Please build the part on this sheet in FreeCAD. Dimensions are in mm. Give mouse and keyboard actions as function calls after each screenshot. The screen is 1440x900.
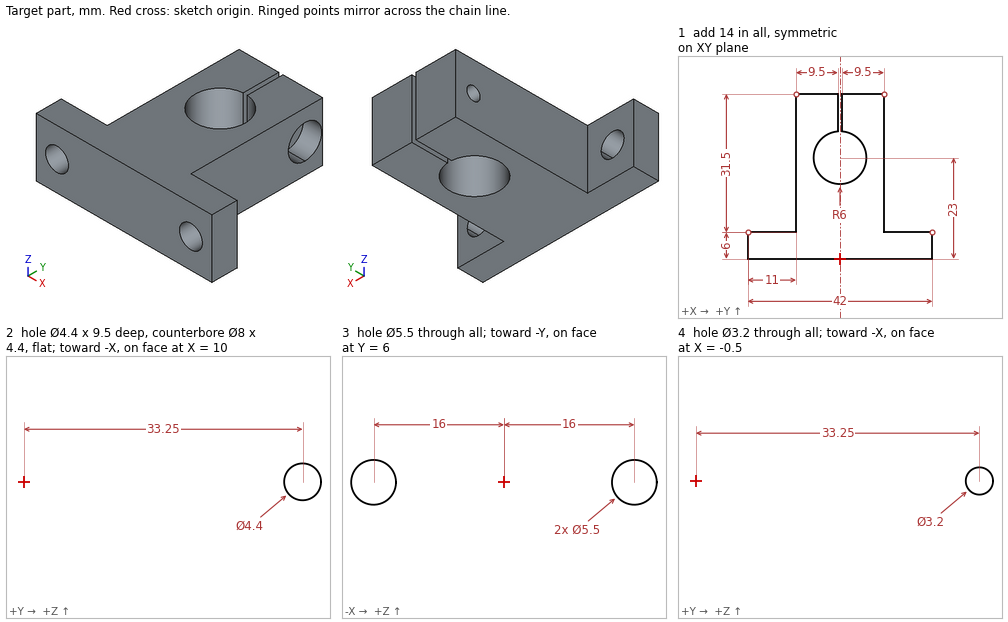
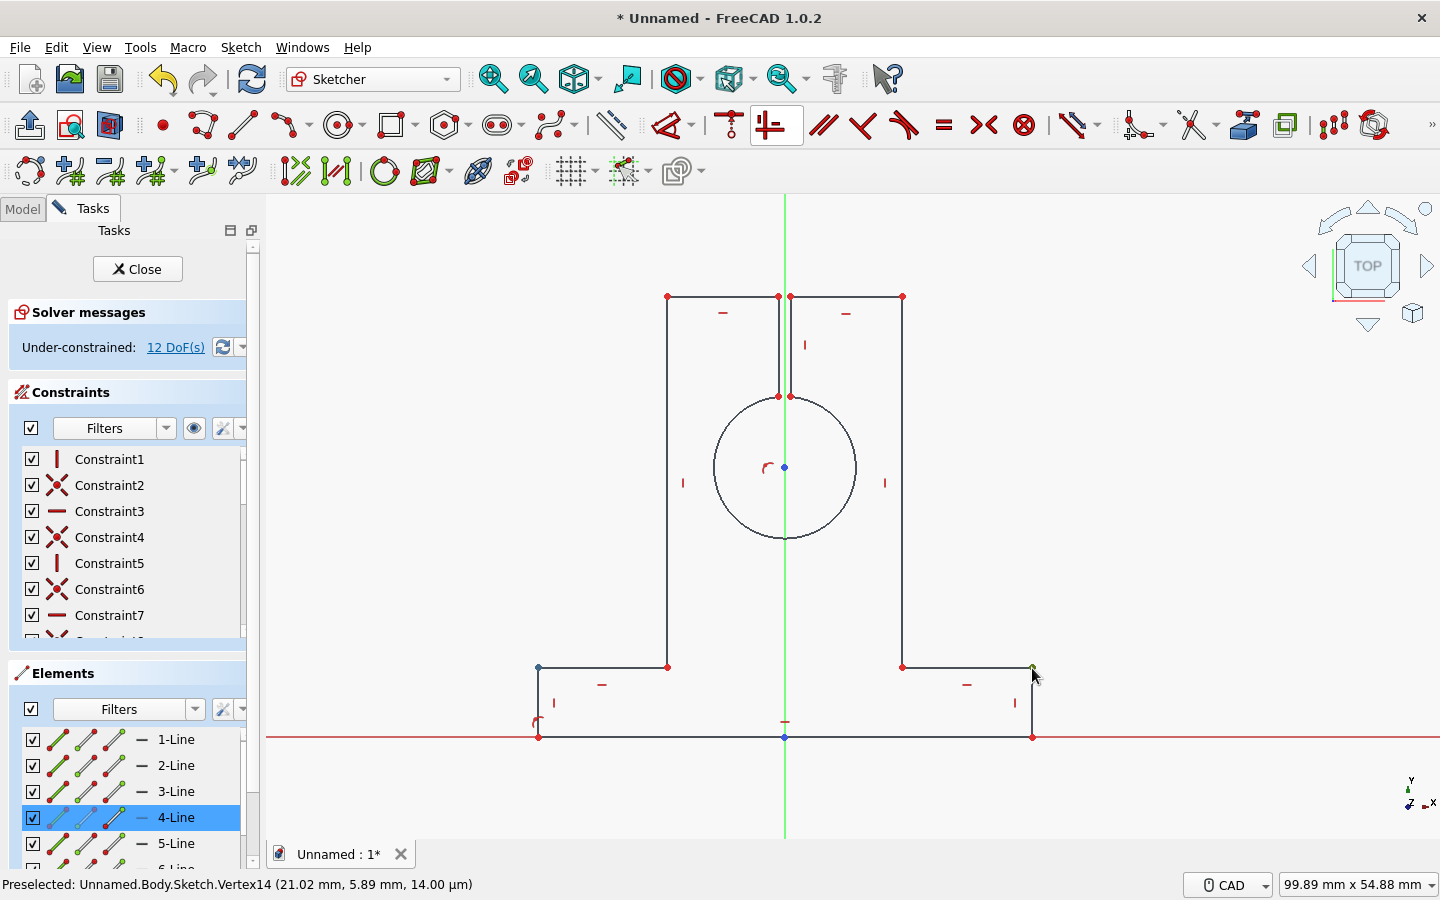
click(785, 769)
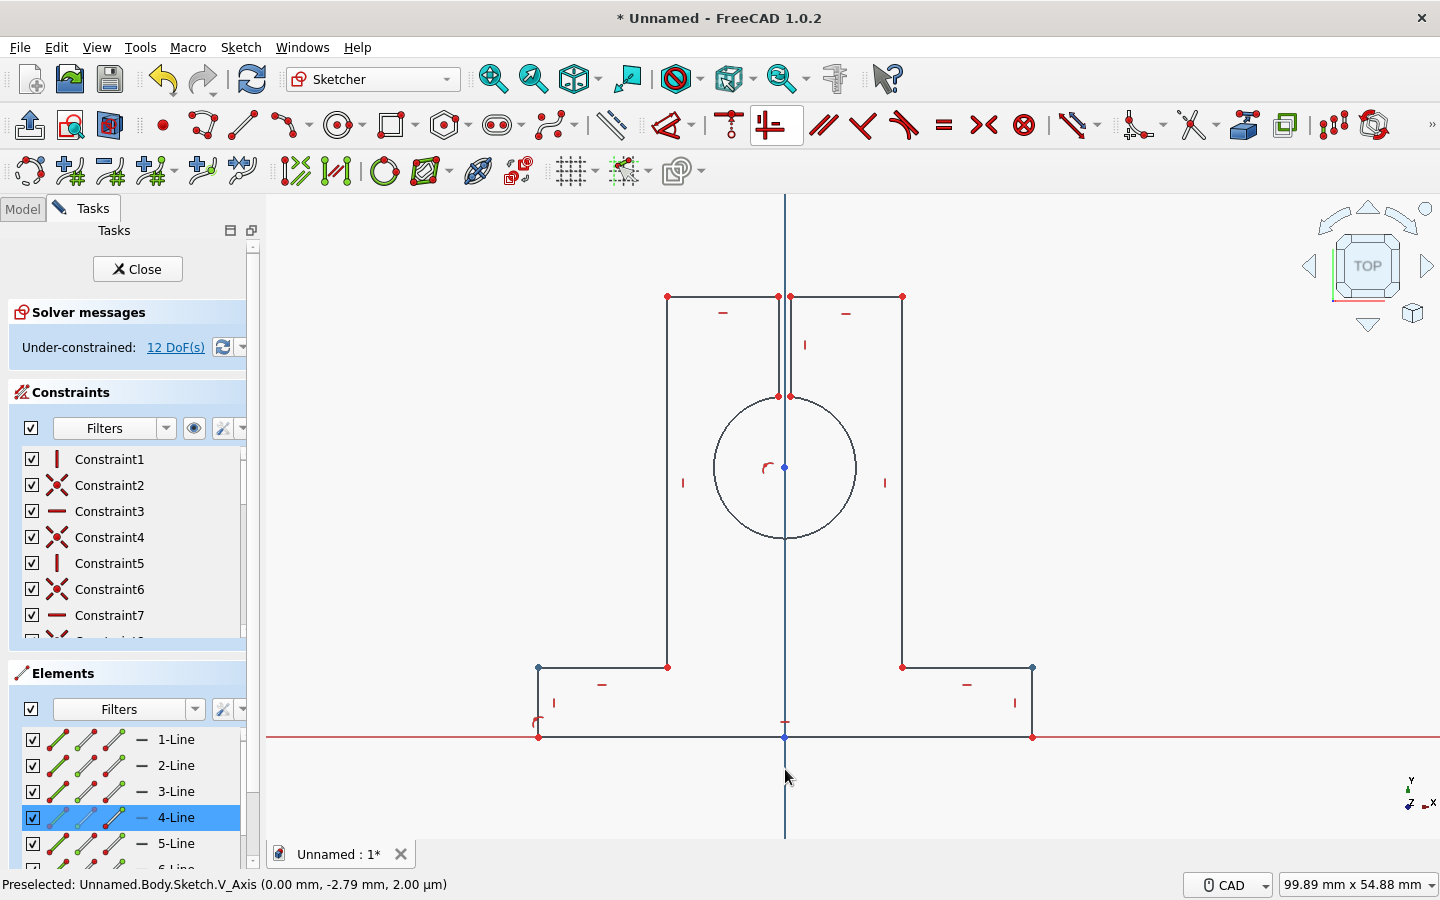
click(984, 126)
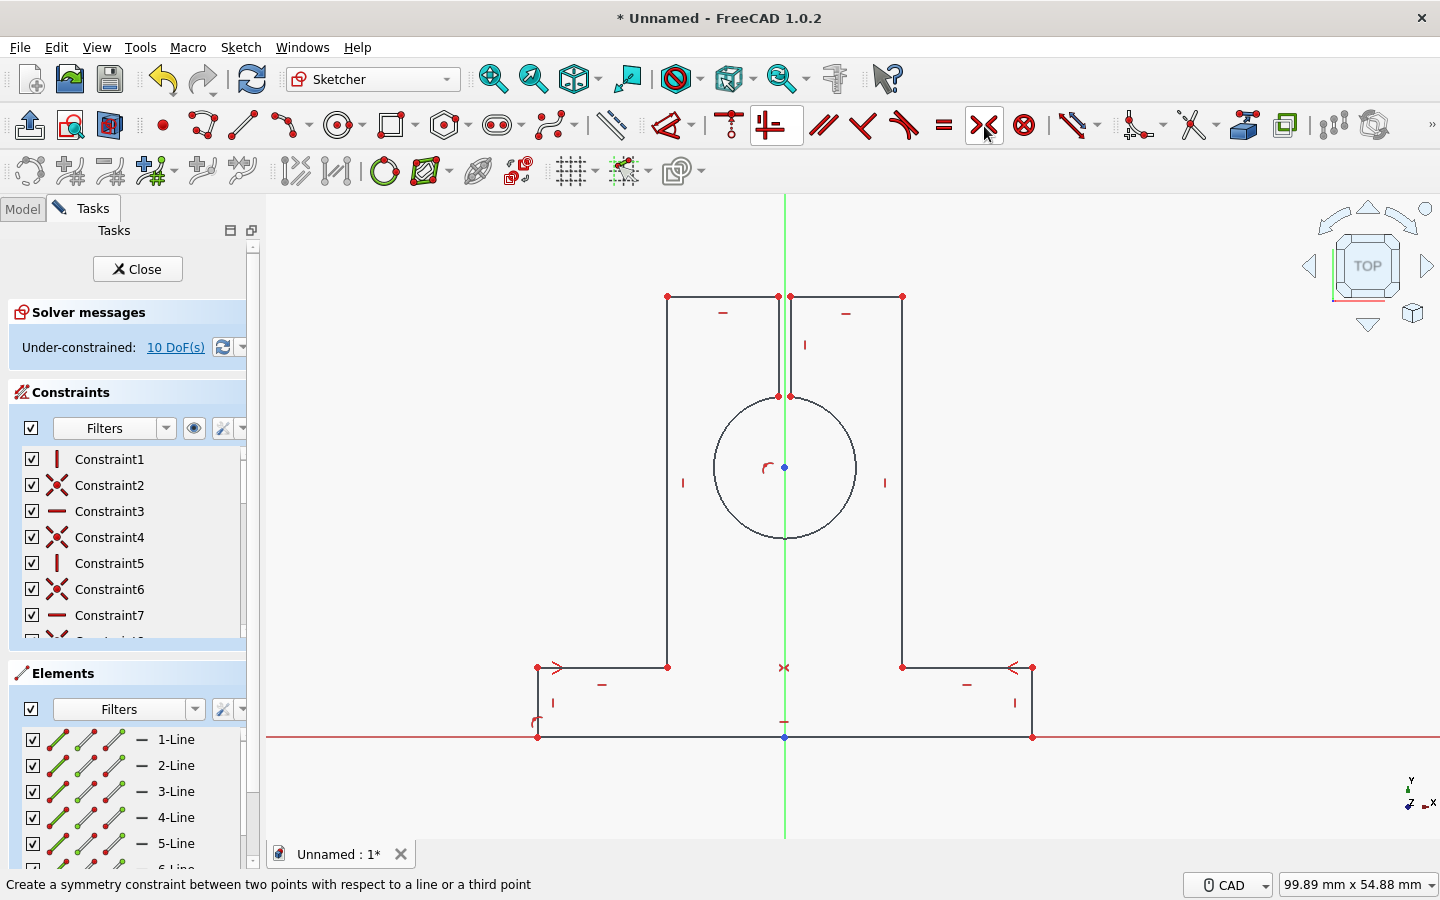
click(667, 297)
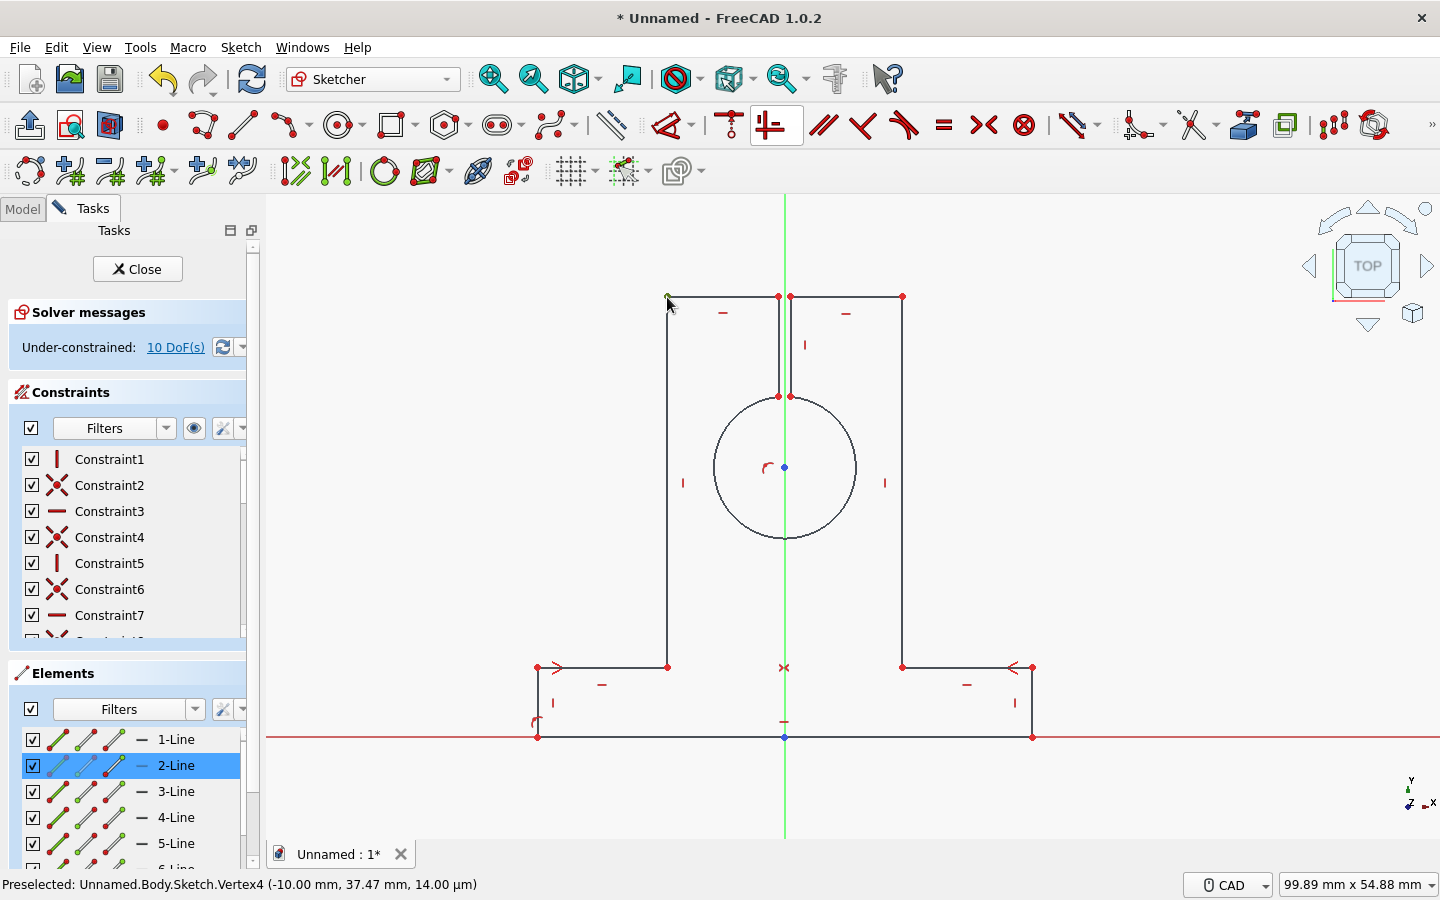
click(902, 297)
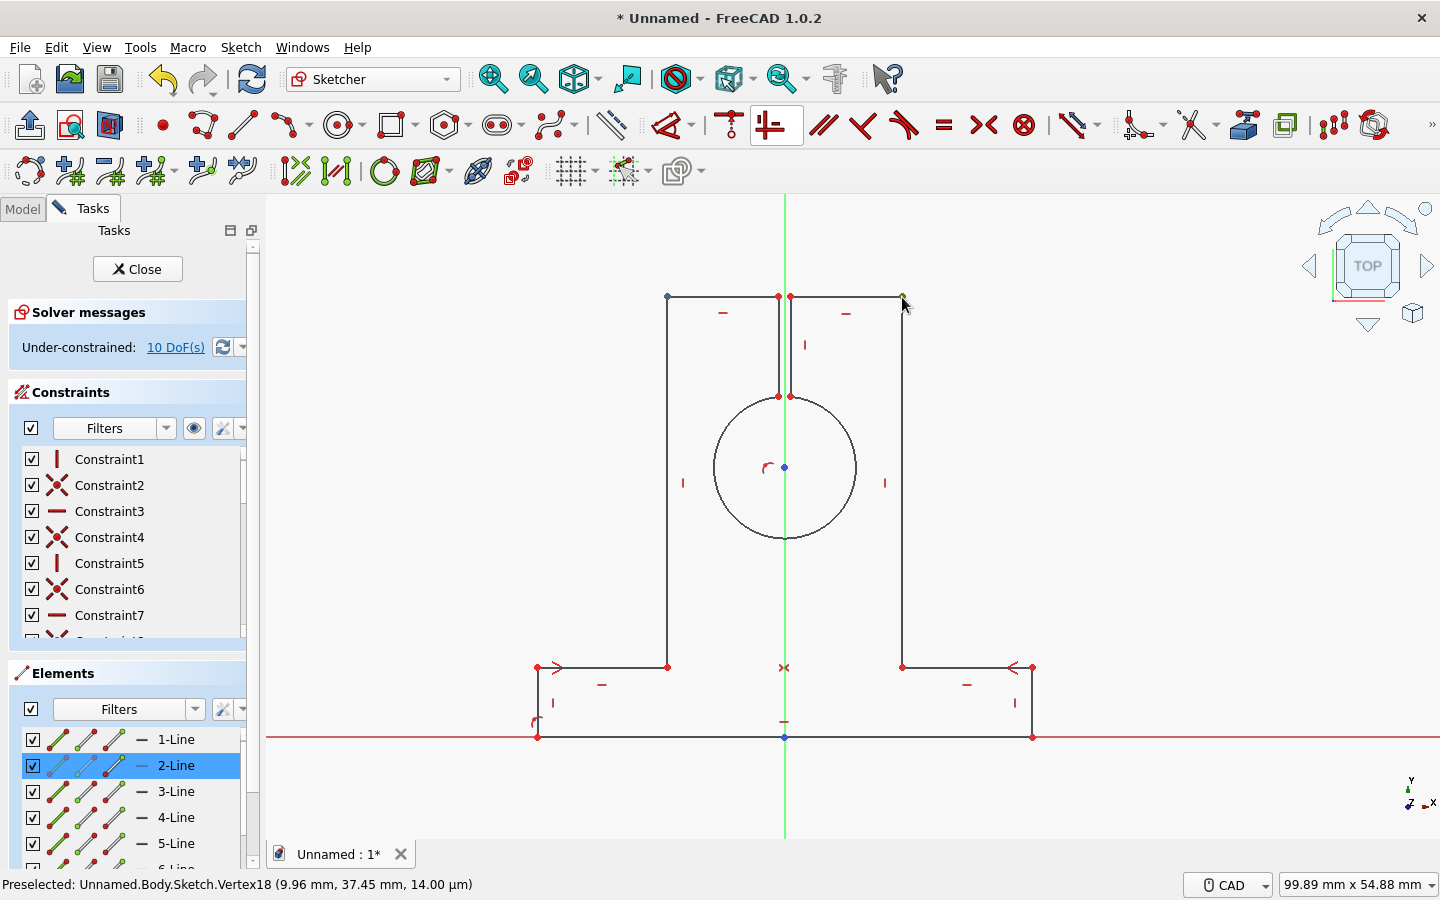
click(785, 769)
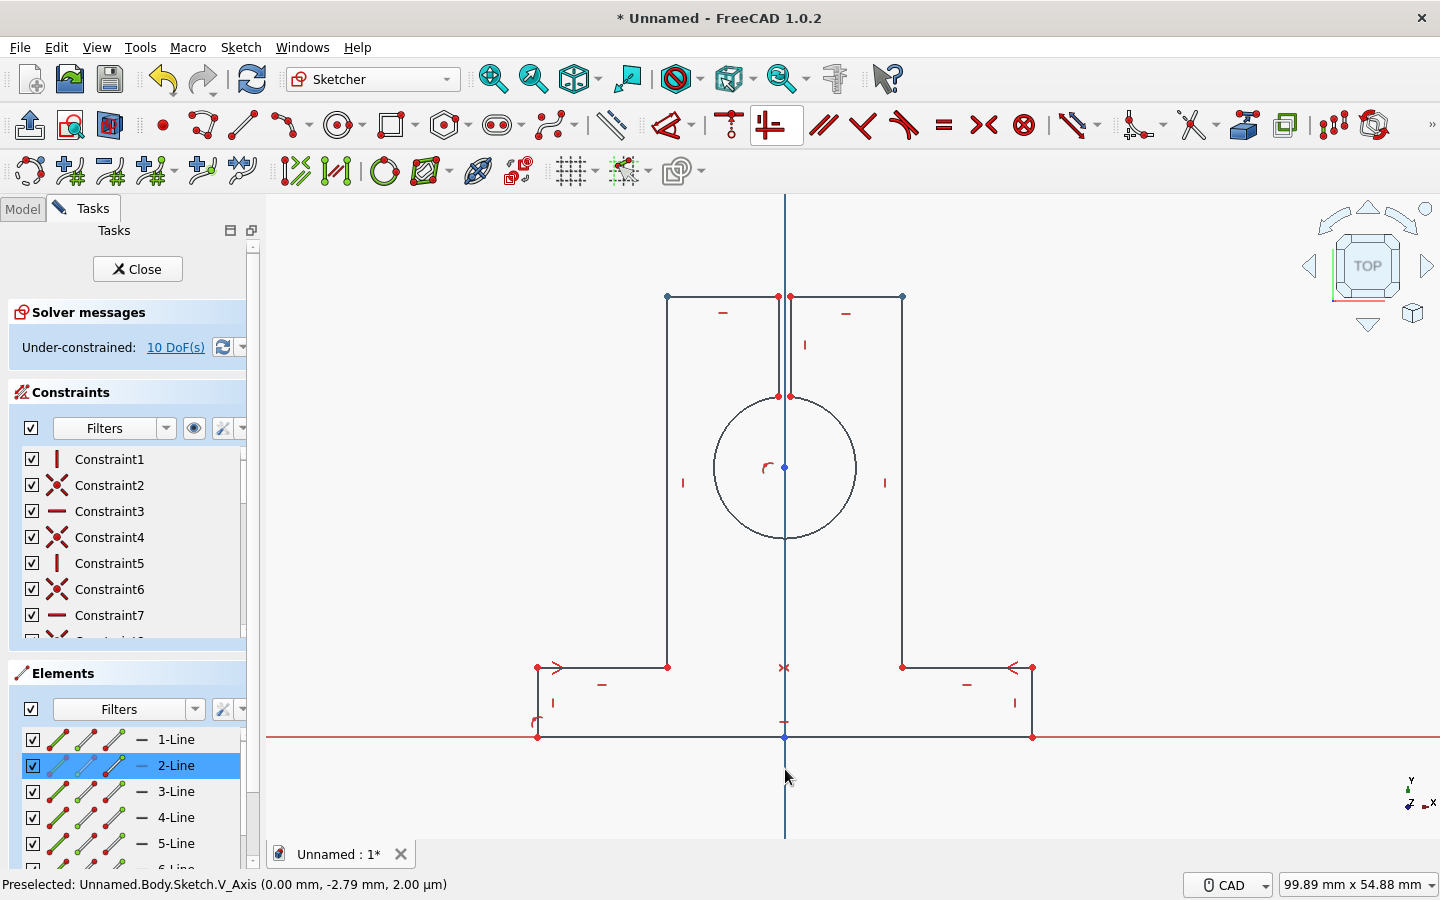
click(984, 126)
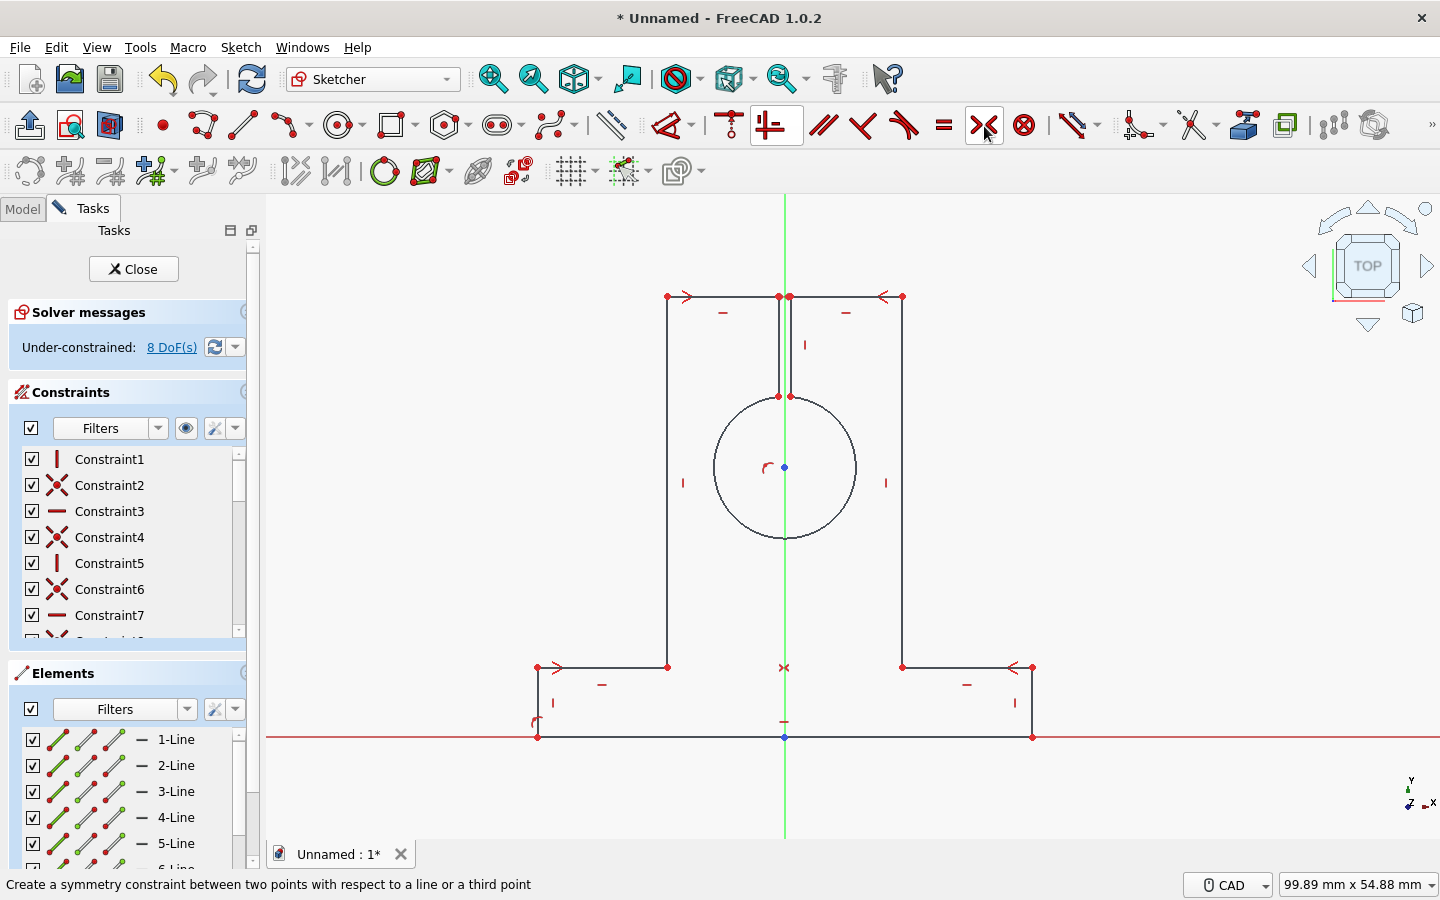
click(718, 492)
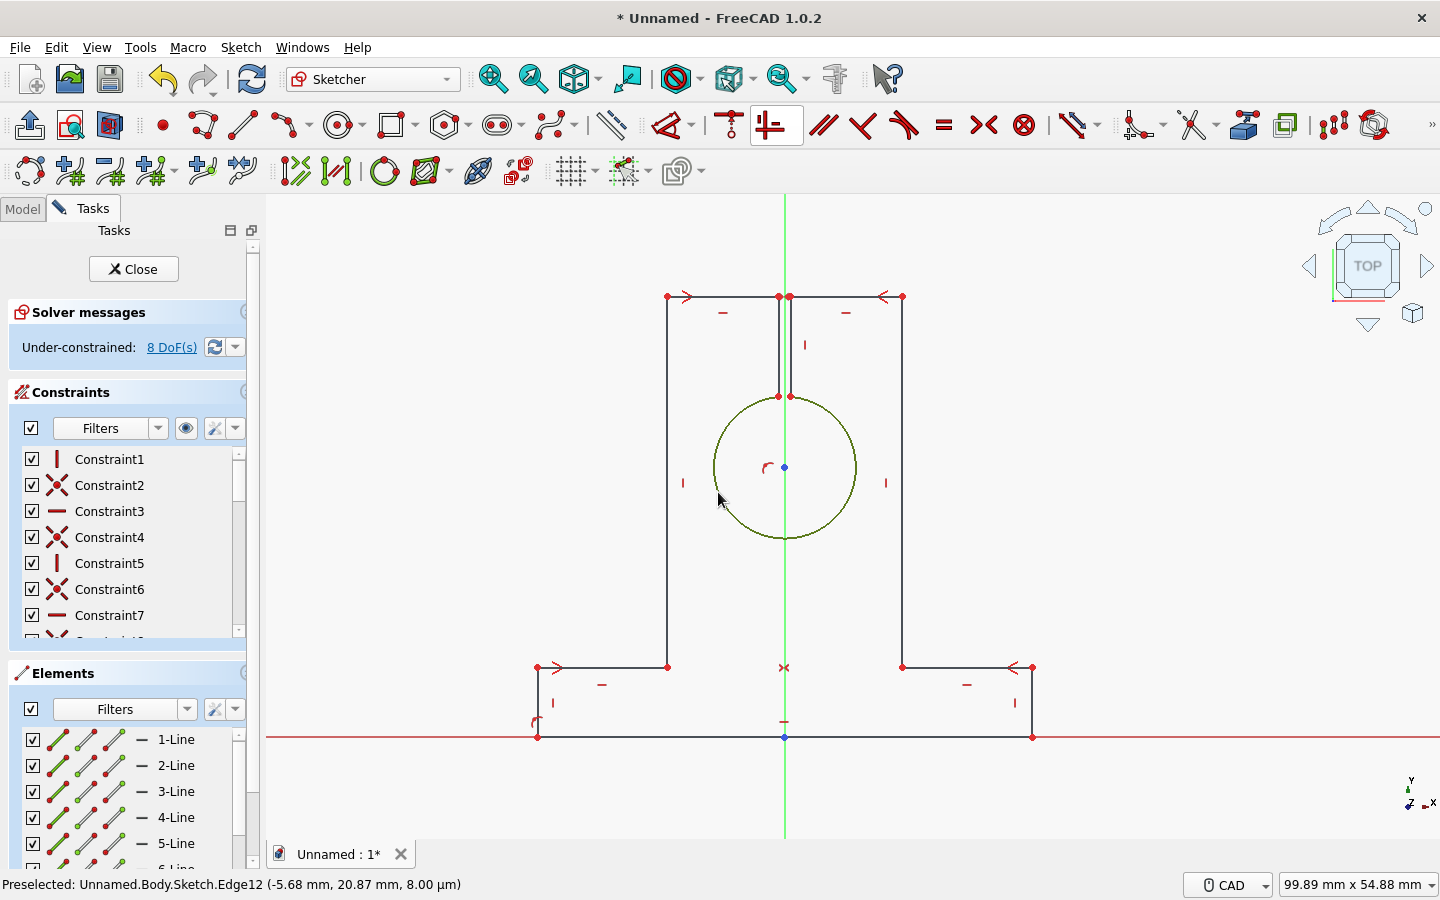
key(k)
key(r)